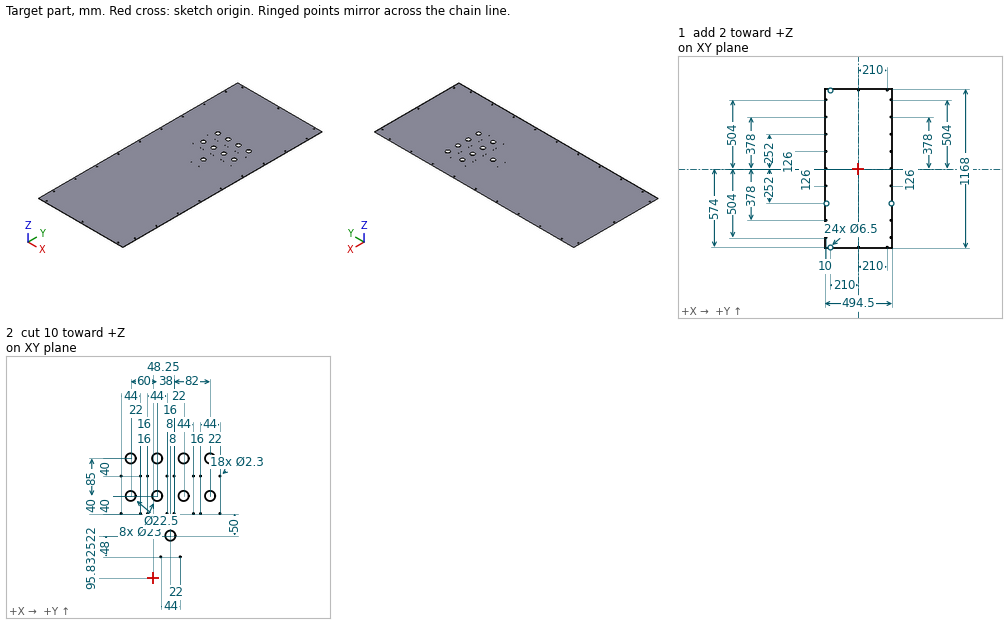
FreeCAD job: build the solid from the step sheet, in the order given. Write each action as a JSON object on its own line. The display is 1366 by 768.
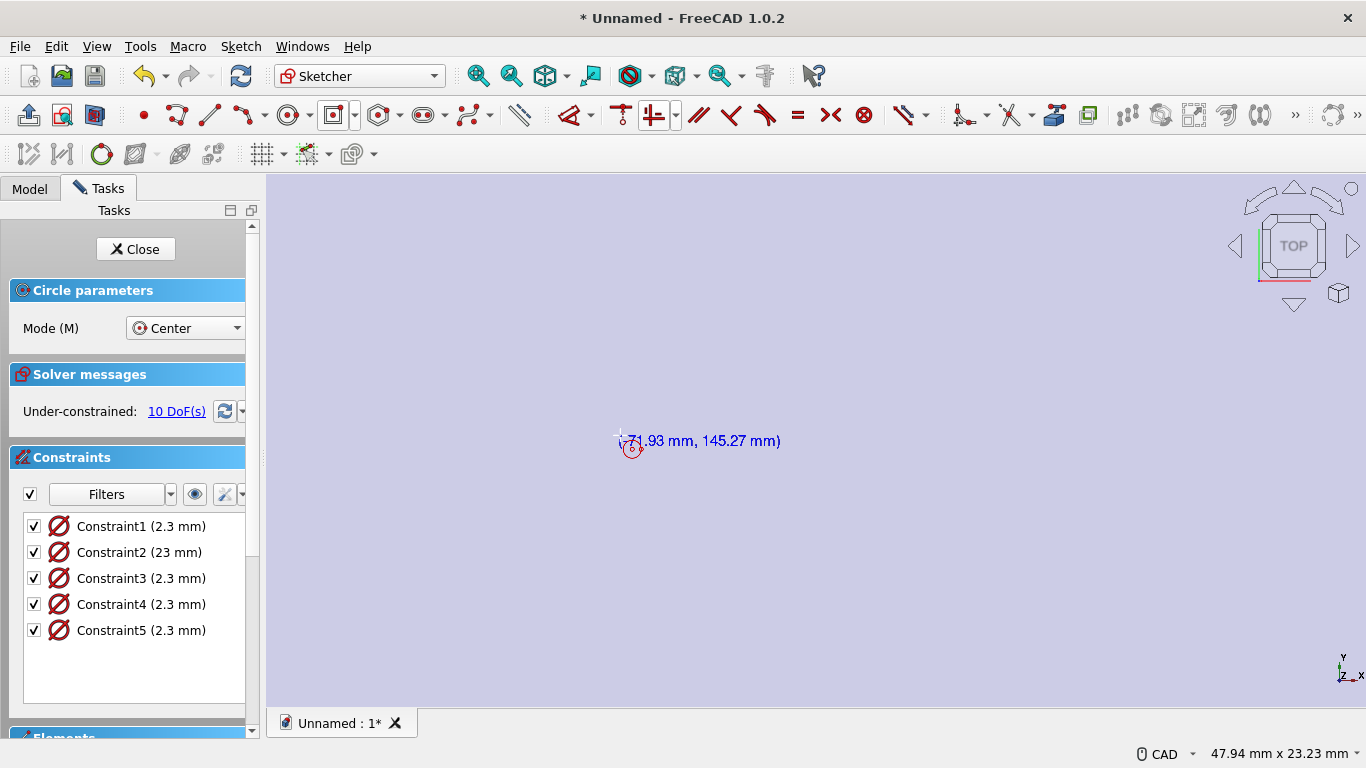
{"action": "scroll", "coordinate": [620, 435], "scroll_direction": "down", "scroll_amount": 15}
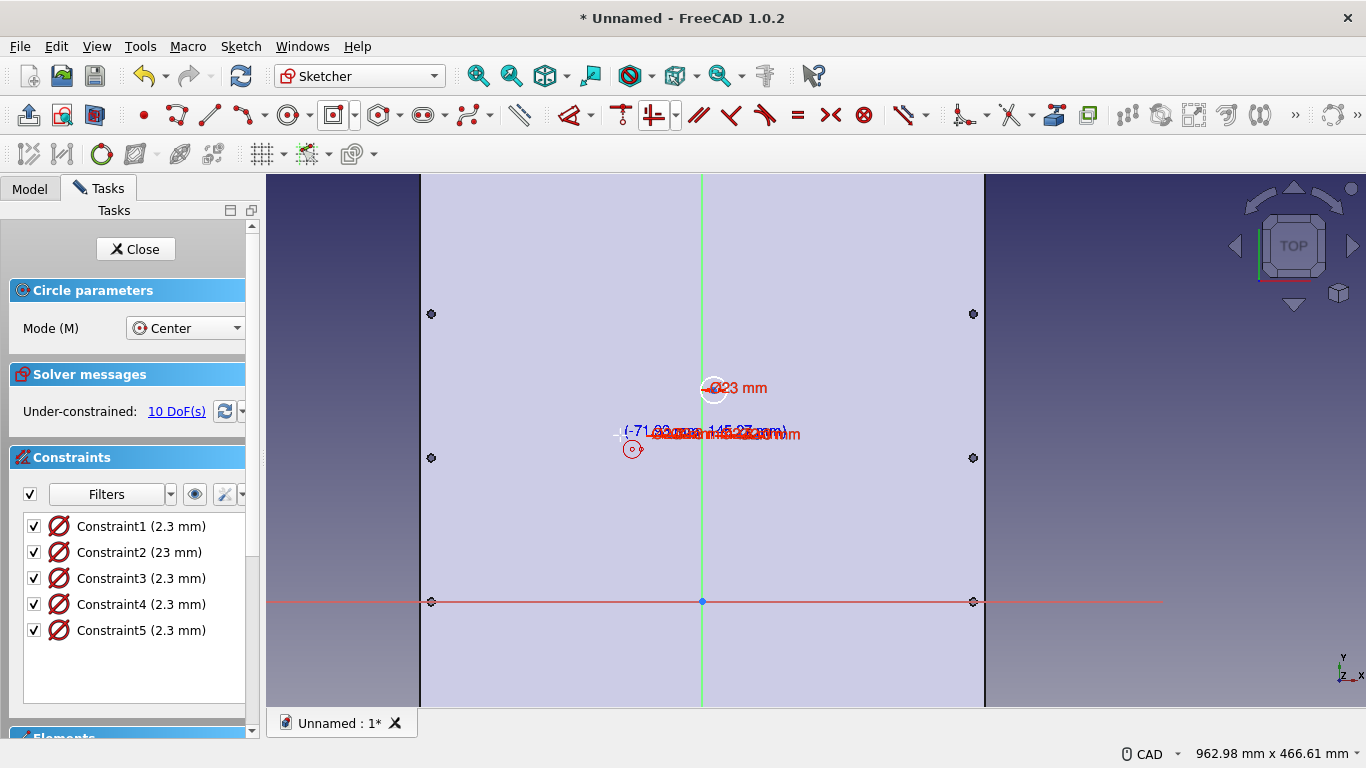
{"action": "left_click", "coordinate": [620, 435]}
{"action": "mouse_move", "coordinate": [621, 434]}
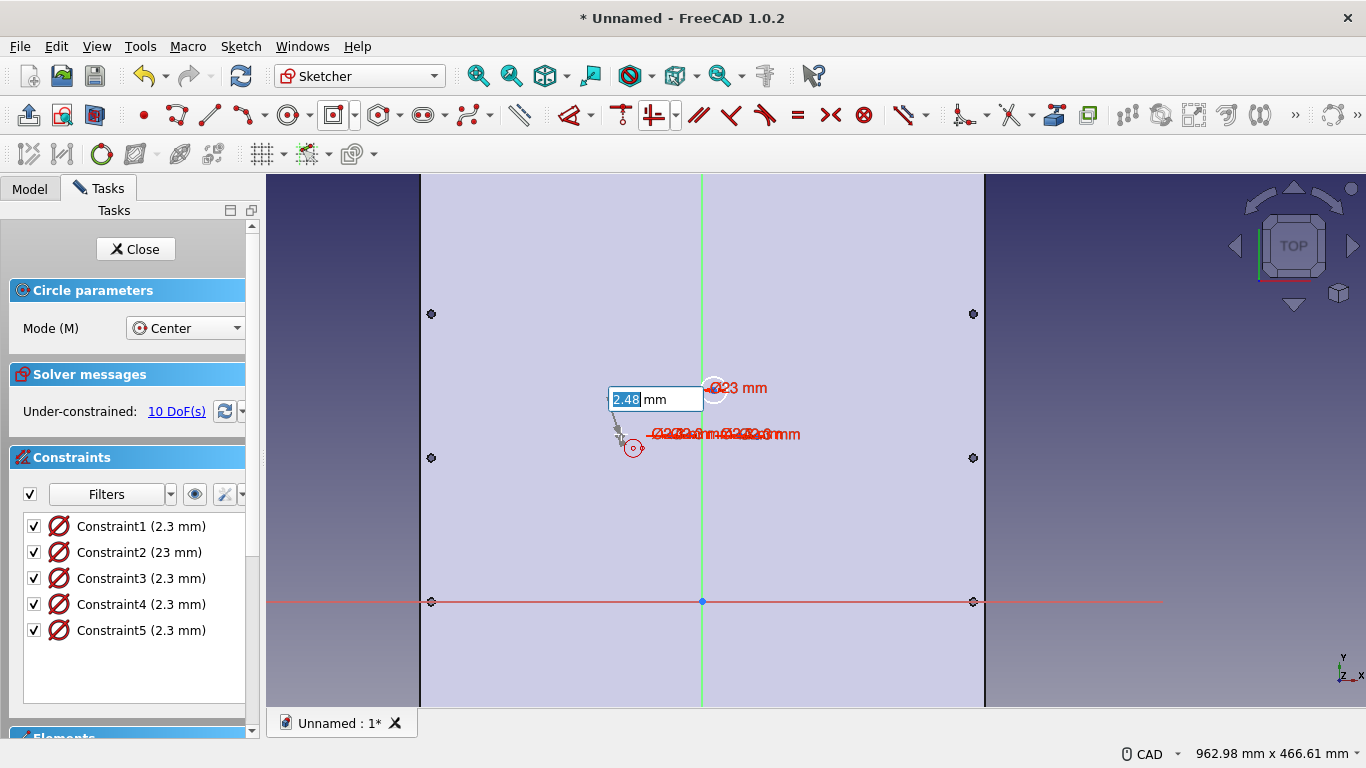
{"action": "type", "text": "2.3"}
{"action": "key", "text": "Return"}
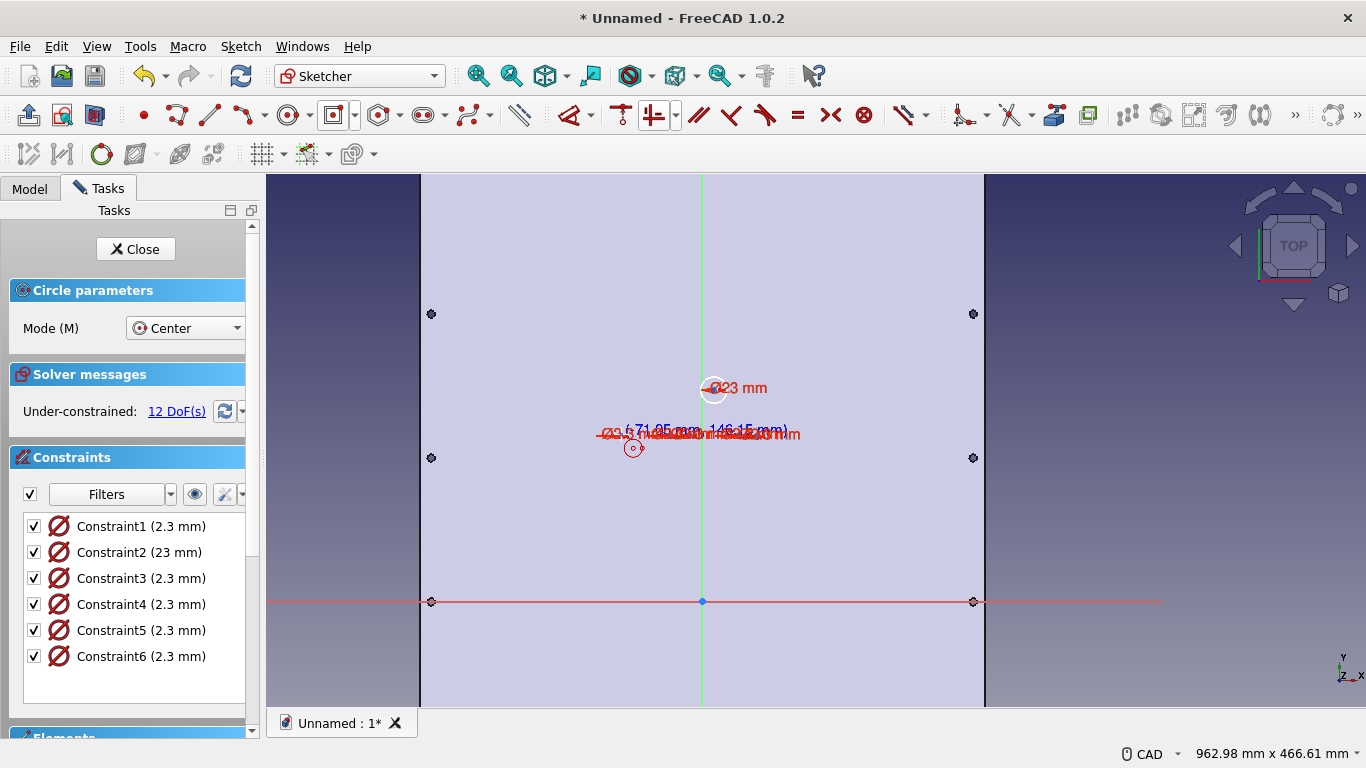
{"action": "scroll", "coordinate": [645, 293], "scroll_direction": "up", "scroll_amount": 3}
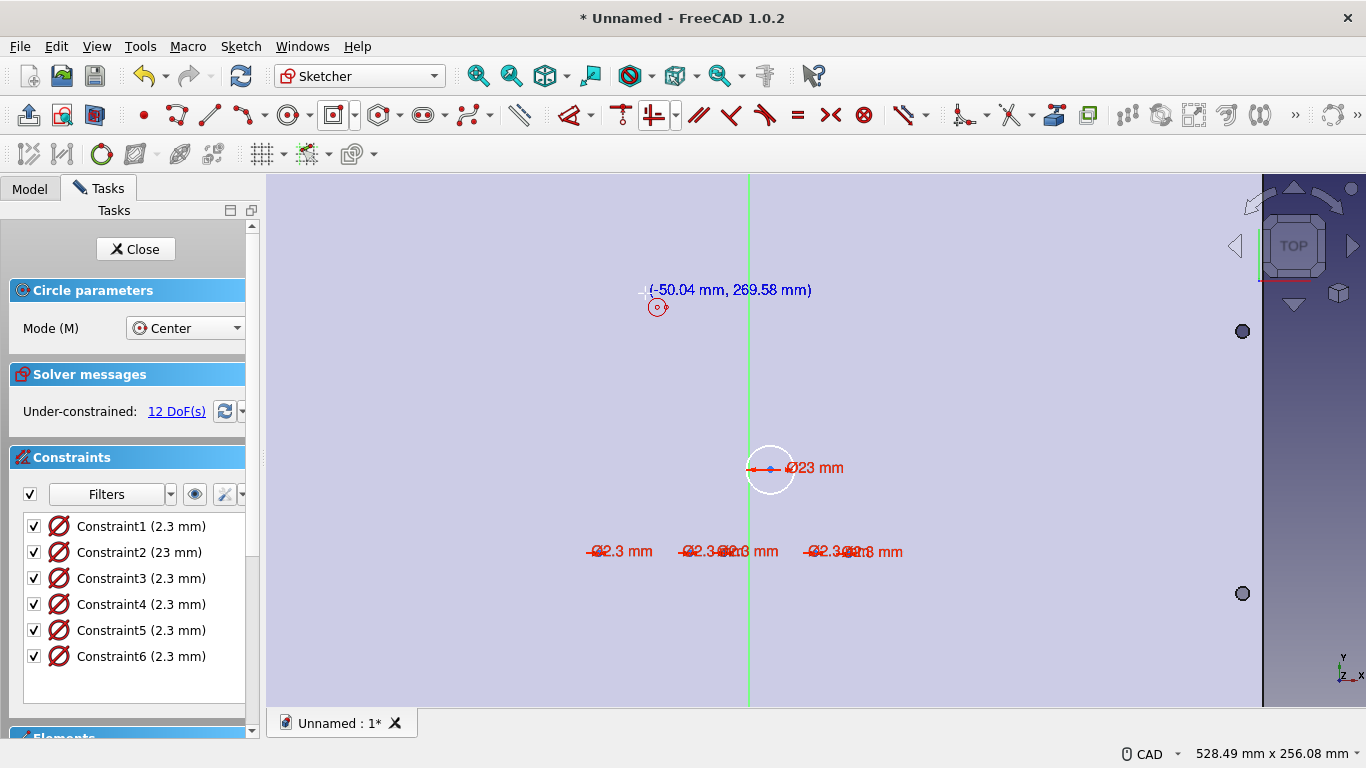
{"action": "left_click", "coordinate": [645, 292]}
{"action": "mouse_move", "coordinate": [662, 275]}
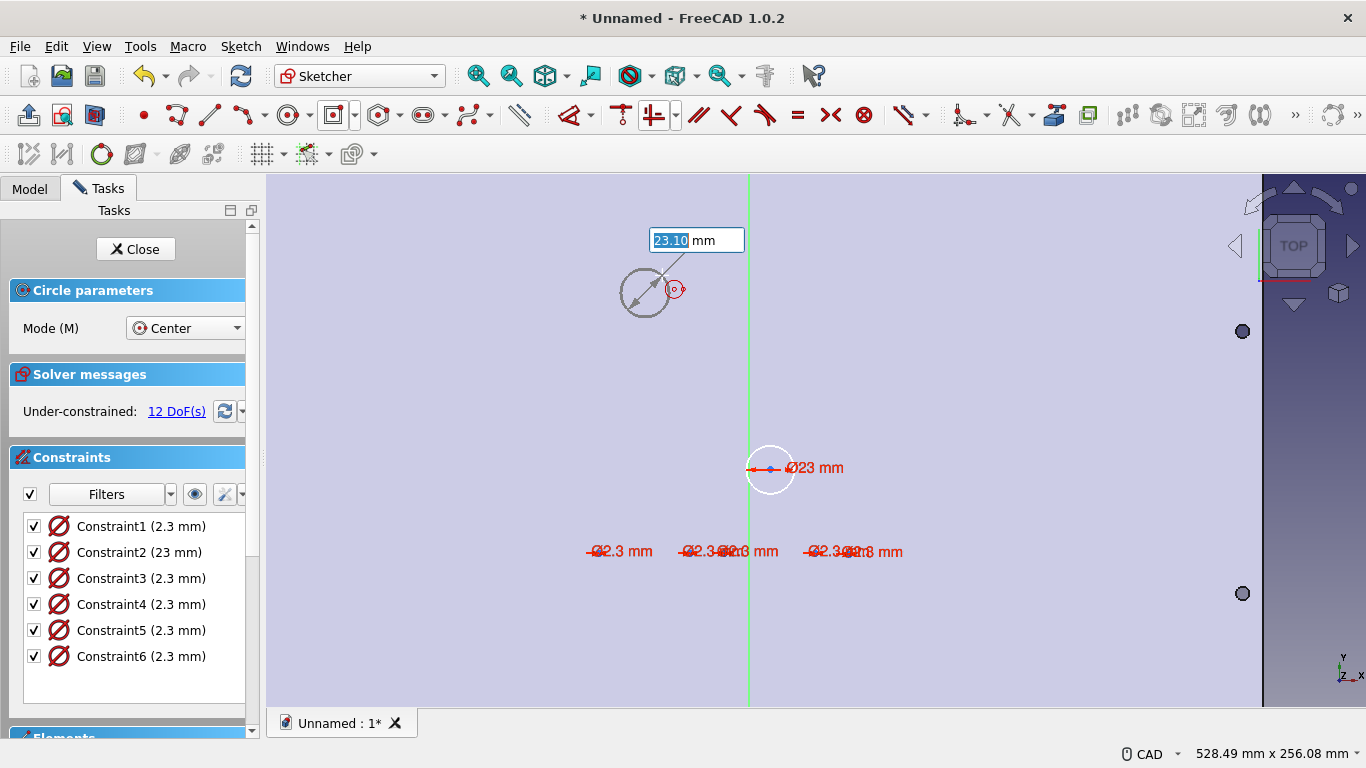
{"action": "type", "text": "23"}
{"action": "key", "text": "Return"}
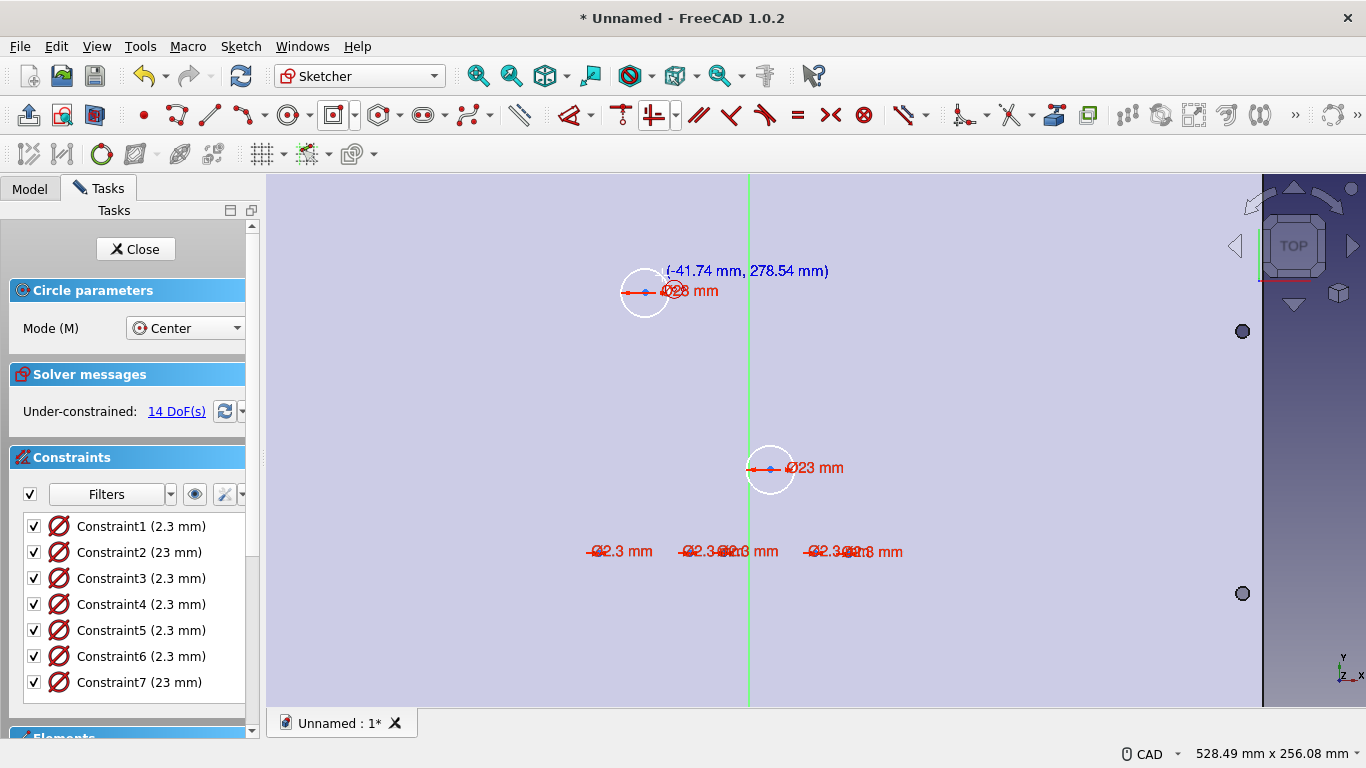
{"action": "scroll", "coordinate": [691, 375], "scroll_direction": "up", "scroll_amount": 12}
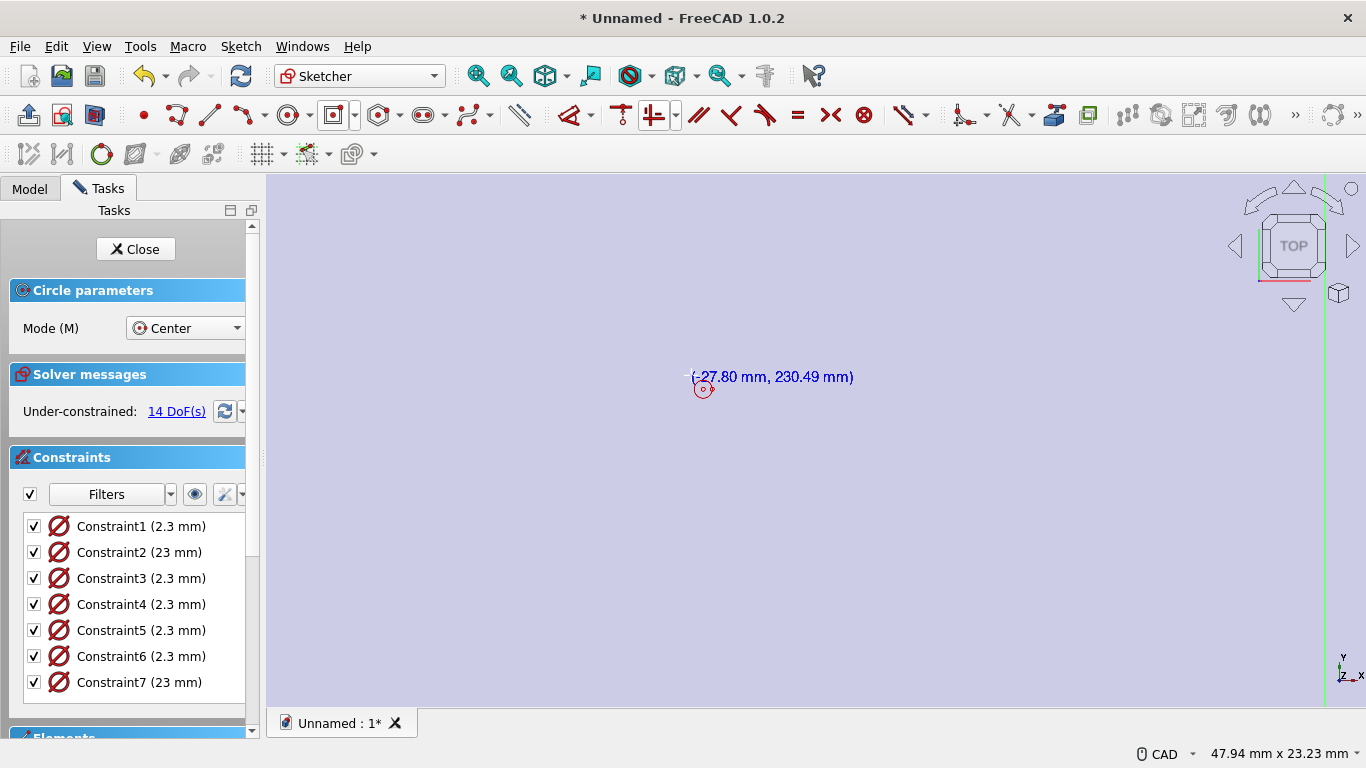
{"action": "scroll", "coordinate": [669, 336], "scroll_direction": "down", "scroll_amount": 15}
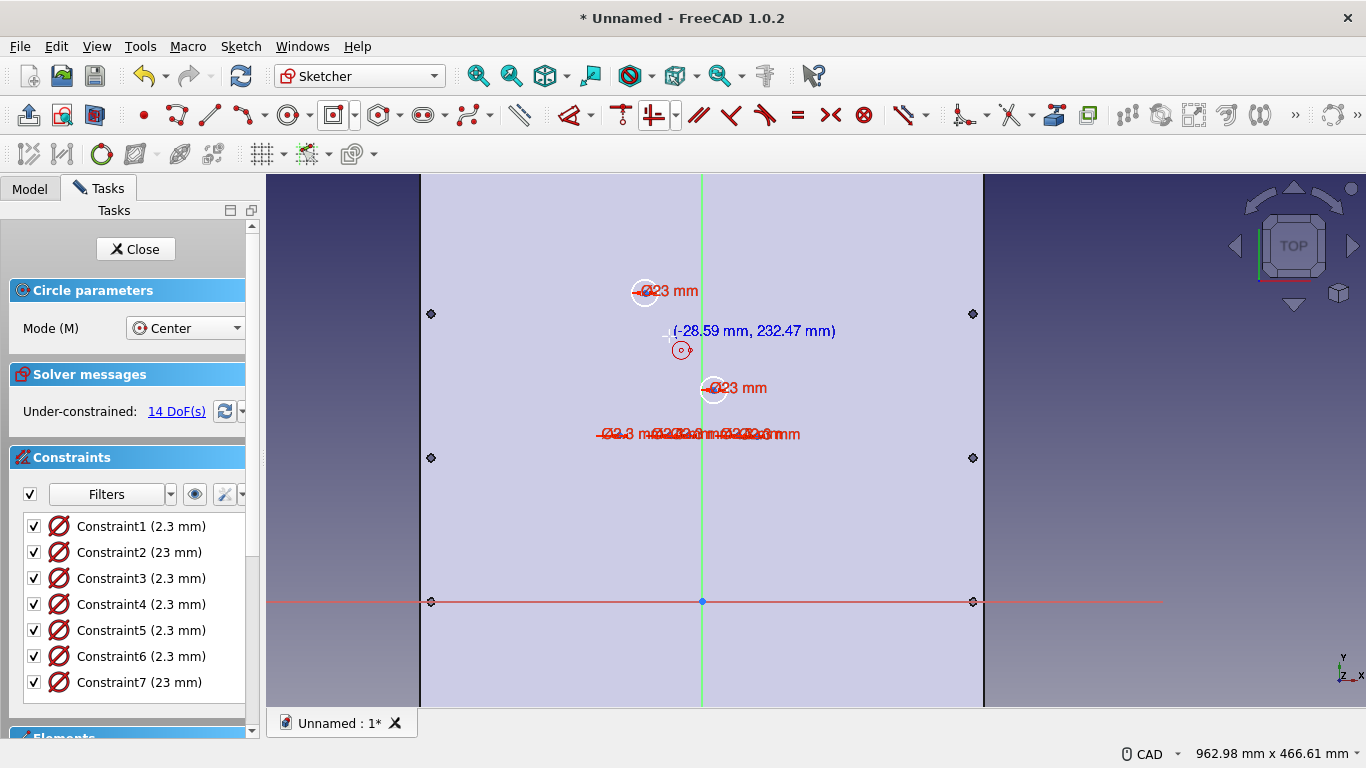
{"action": "left_click", "coordinate": [670, 338]}
{"action": "mouse_move", "coordinate": [671, 337]}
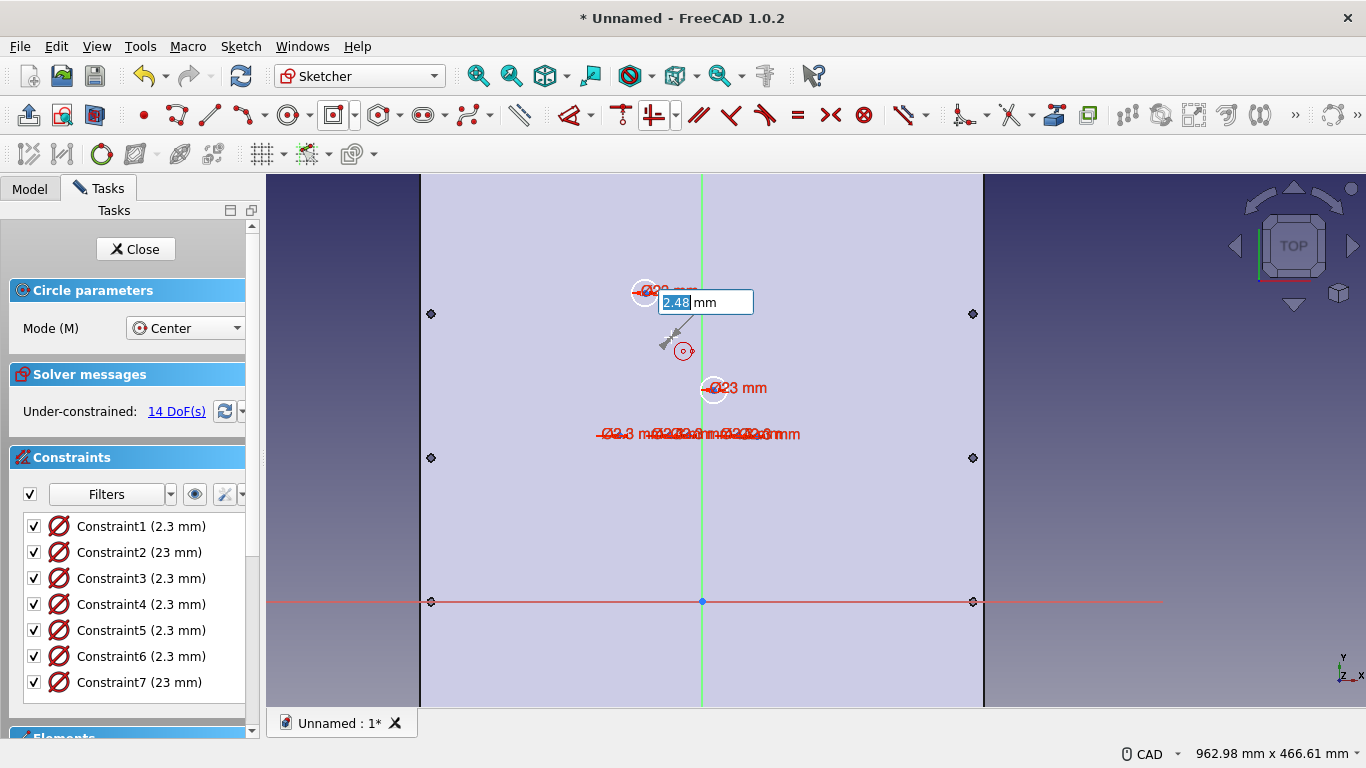
{"action": "type", "text": "2.3"}
{"action": "key", "text": "Return"}